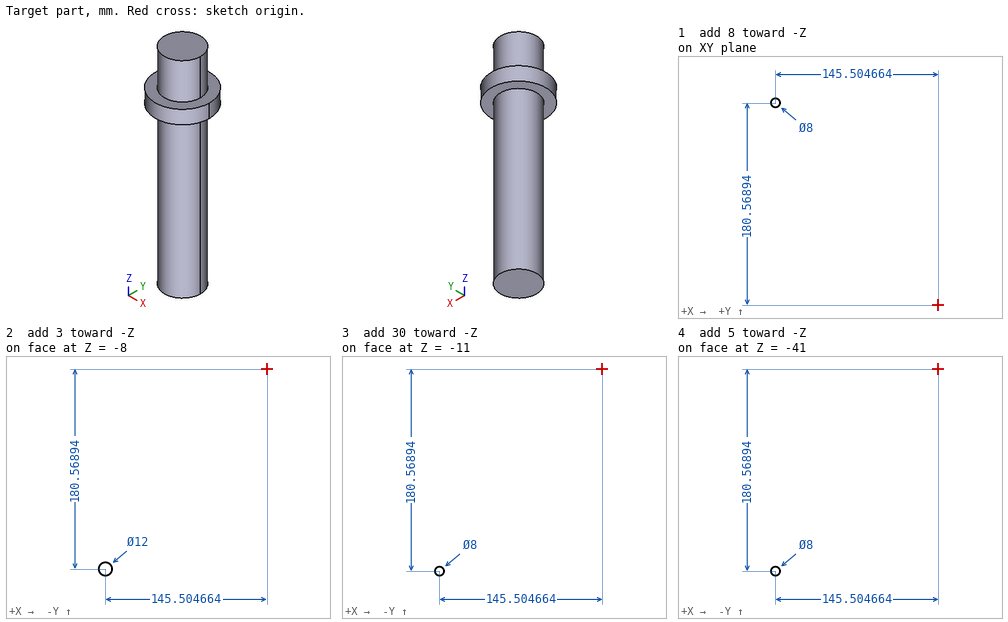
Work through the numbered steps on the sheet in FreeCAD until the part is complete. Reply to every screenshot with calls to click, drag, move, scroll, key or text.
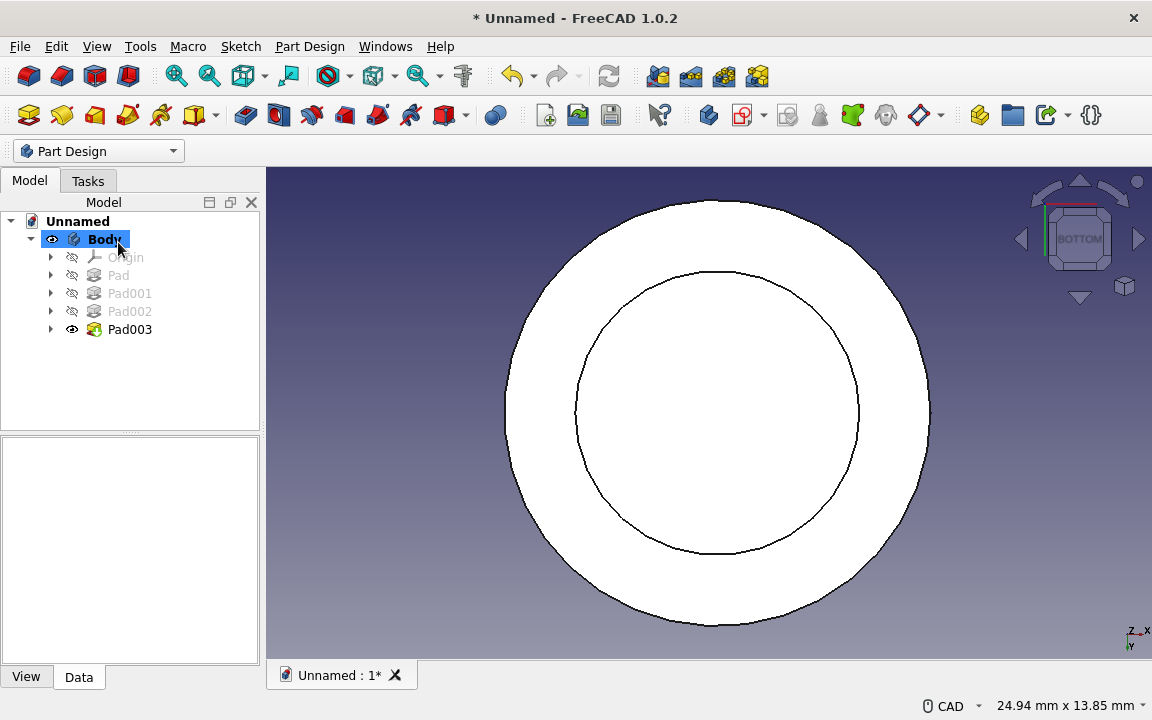
key(0)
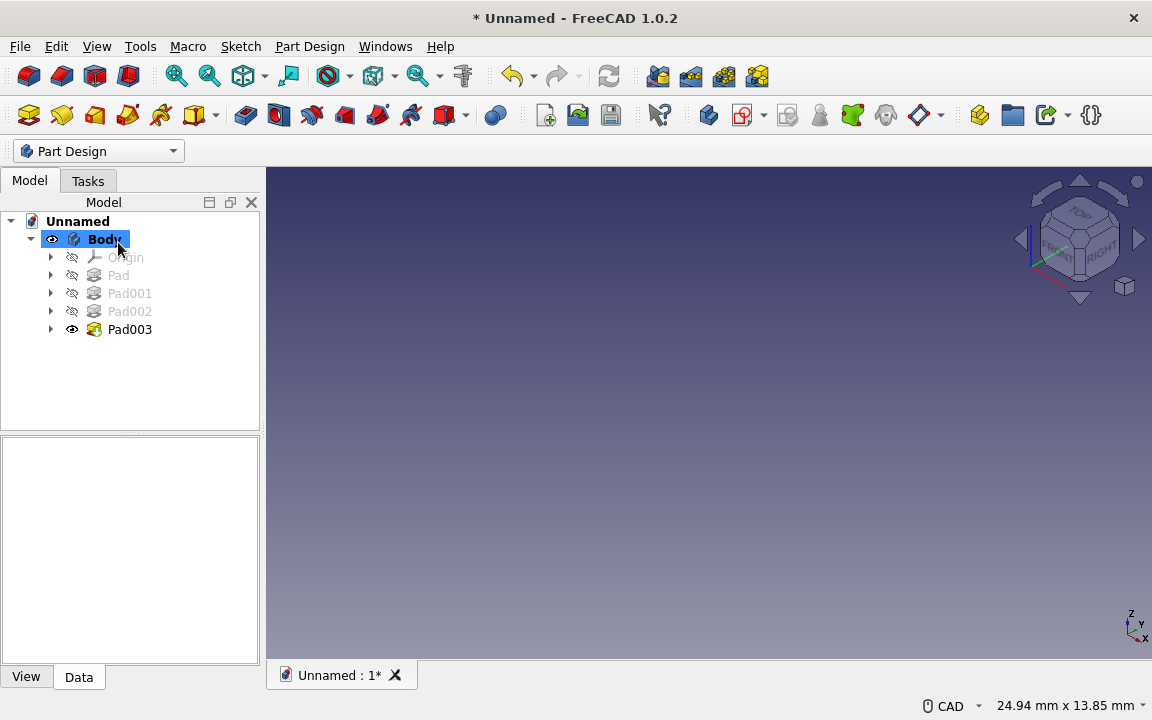
click(177, 76)